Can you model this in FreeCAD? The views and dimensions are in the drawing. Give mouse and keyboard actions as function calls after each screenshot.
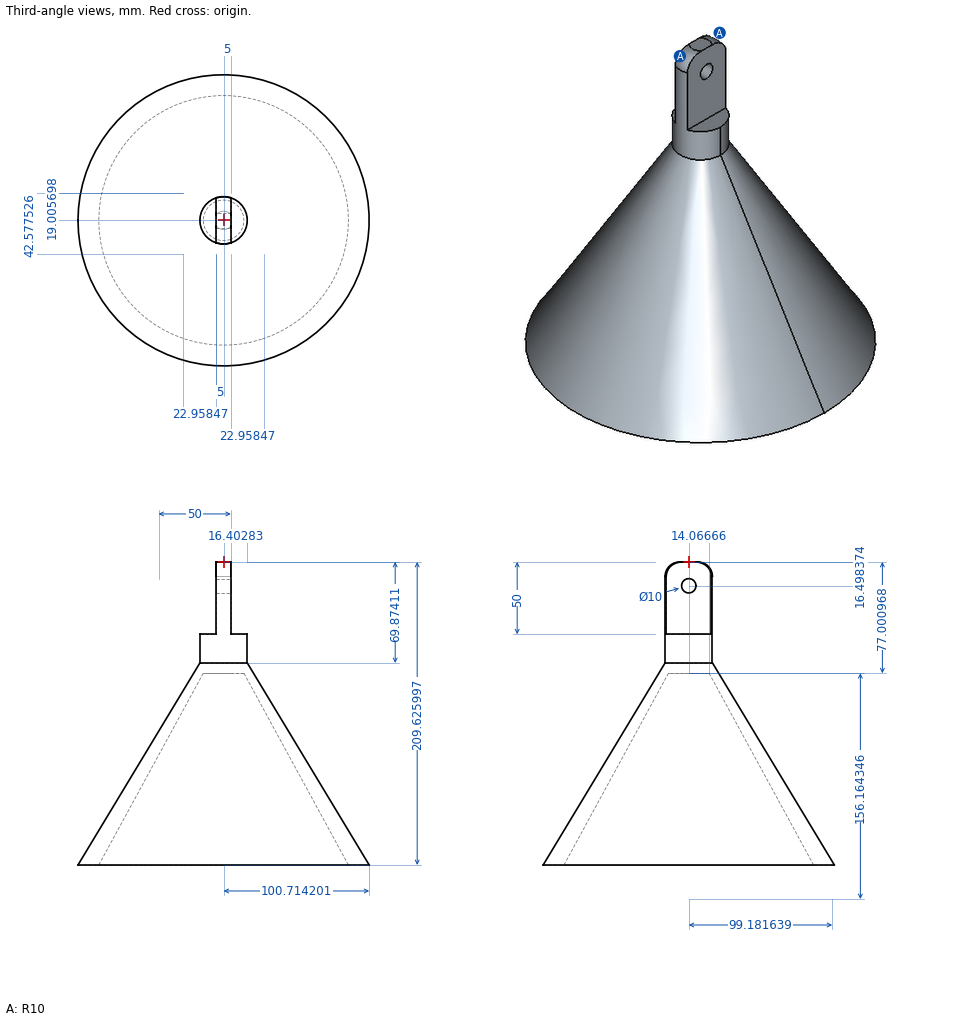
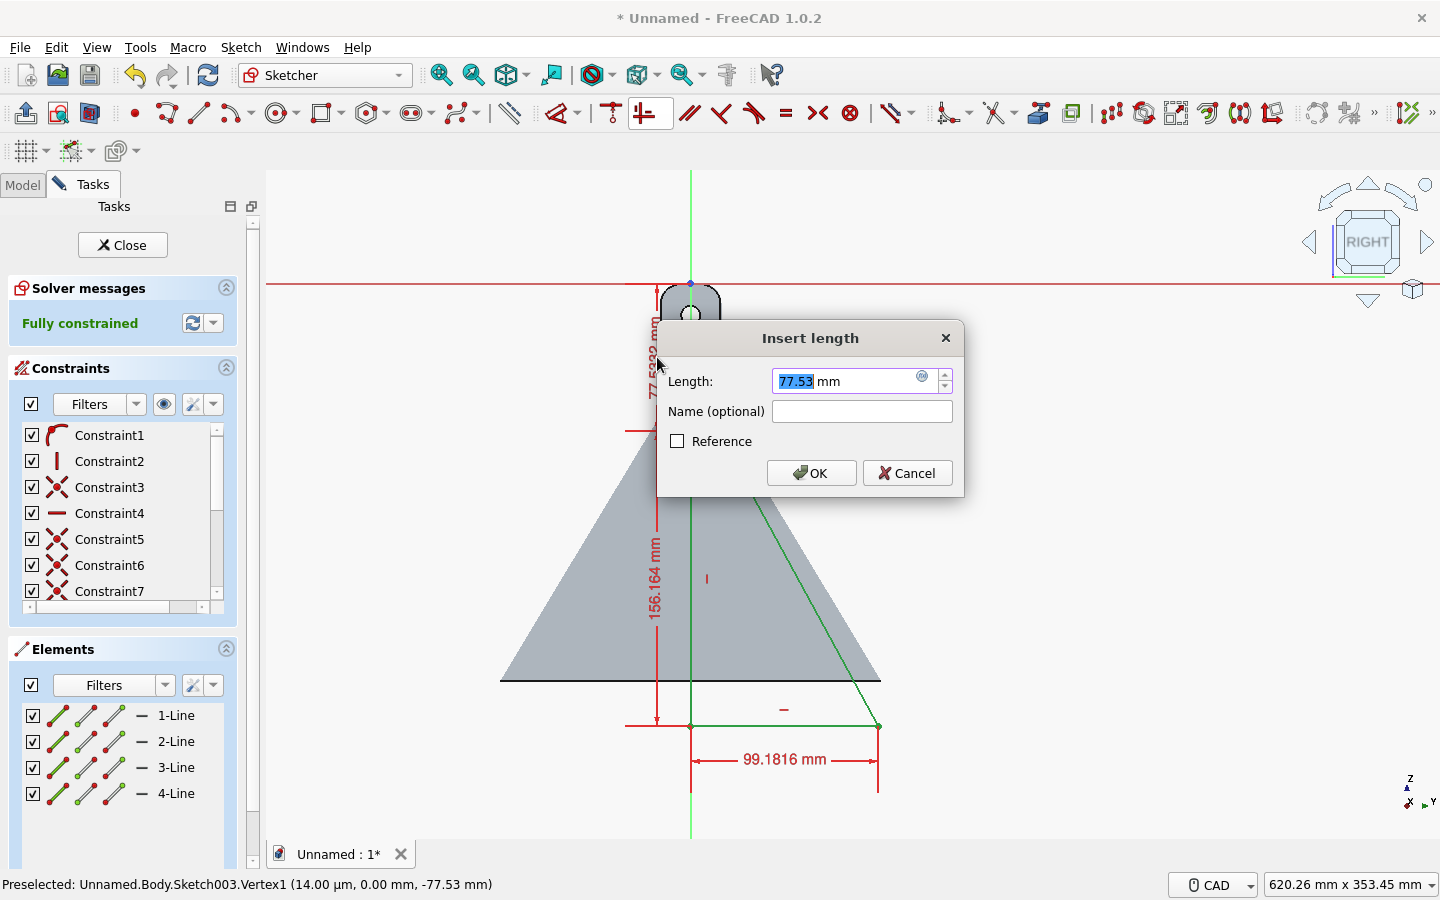
text(77.000968)
key(Return)
key(Escape)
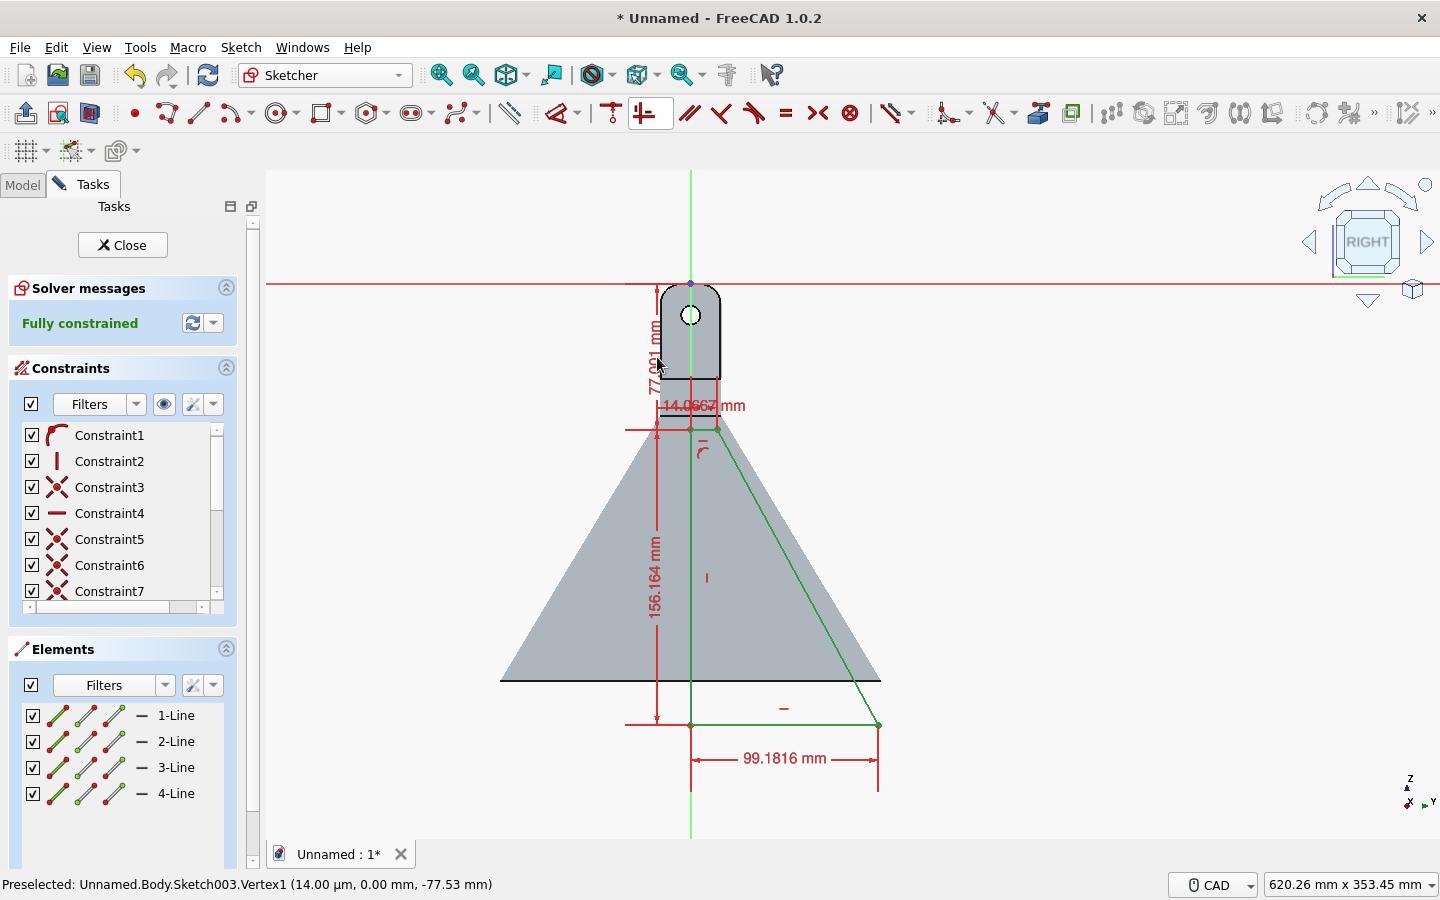
click(123, 245)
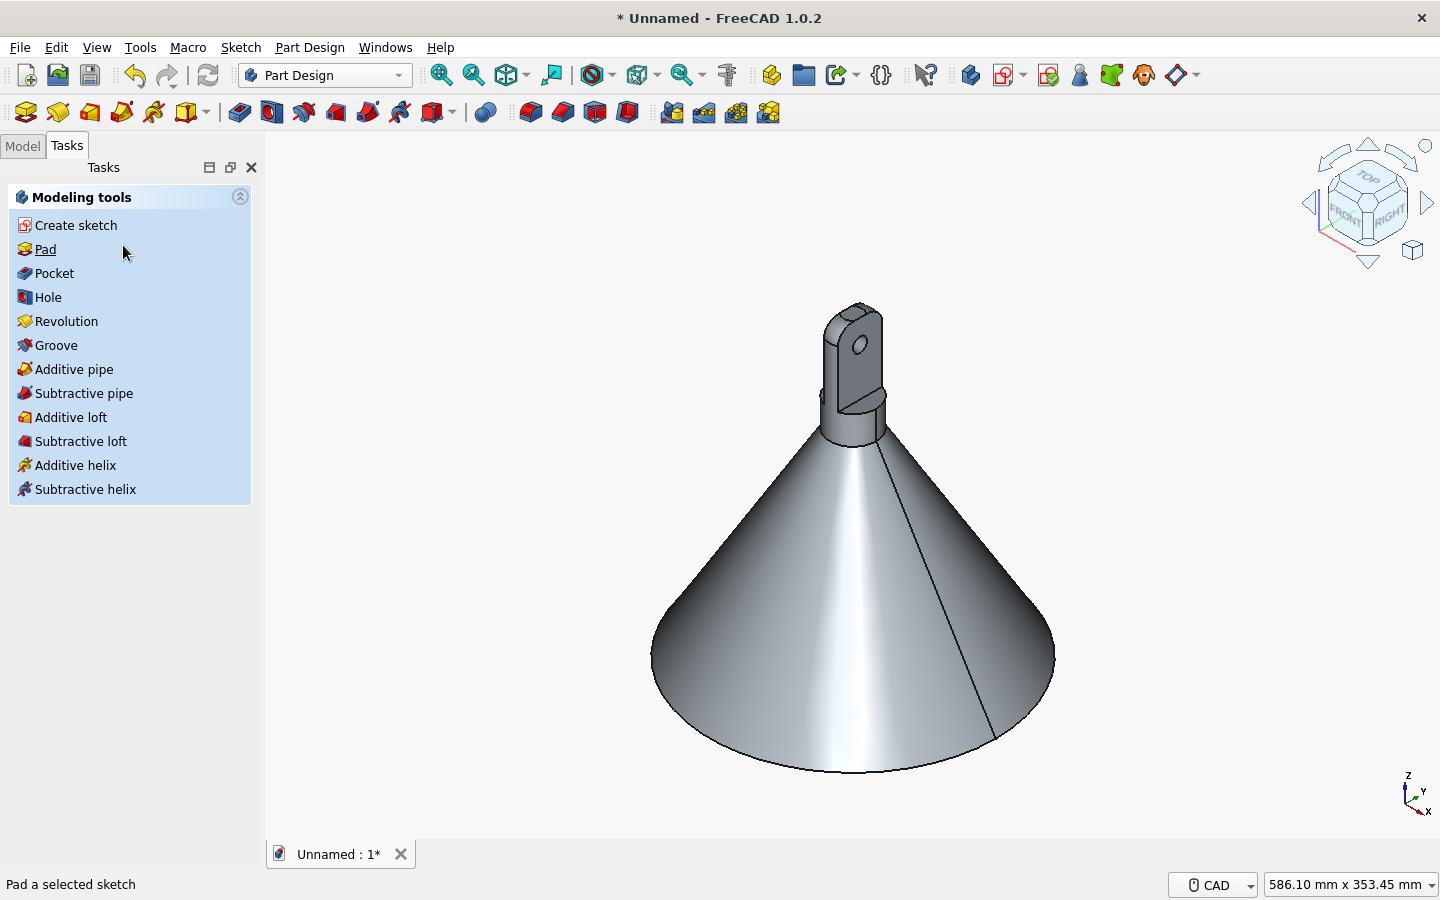
click(304, 112)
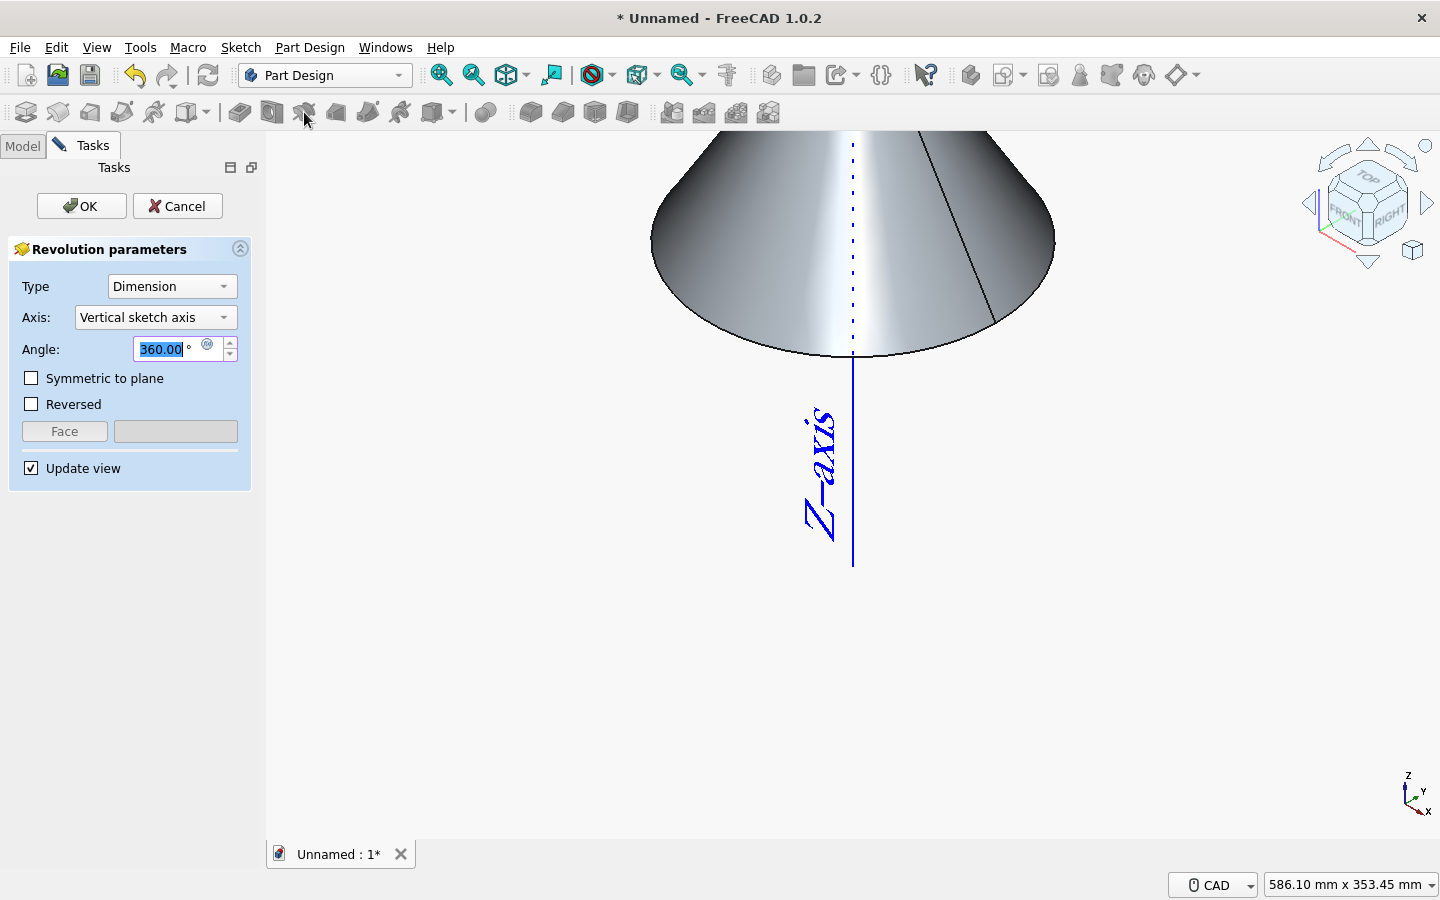
click(82, 206)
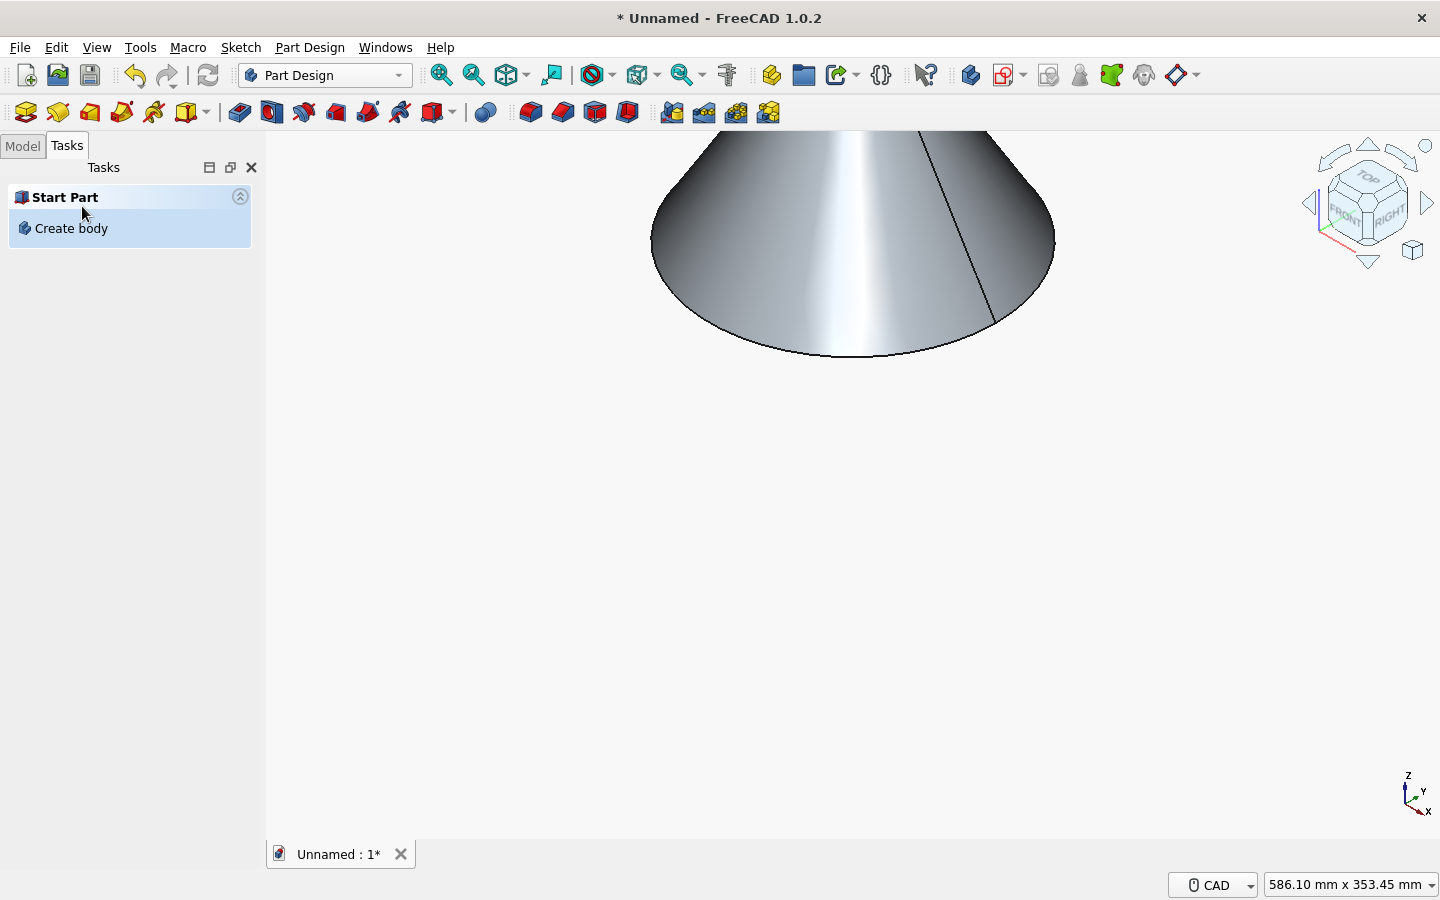
click(442, 76)